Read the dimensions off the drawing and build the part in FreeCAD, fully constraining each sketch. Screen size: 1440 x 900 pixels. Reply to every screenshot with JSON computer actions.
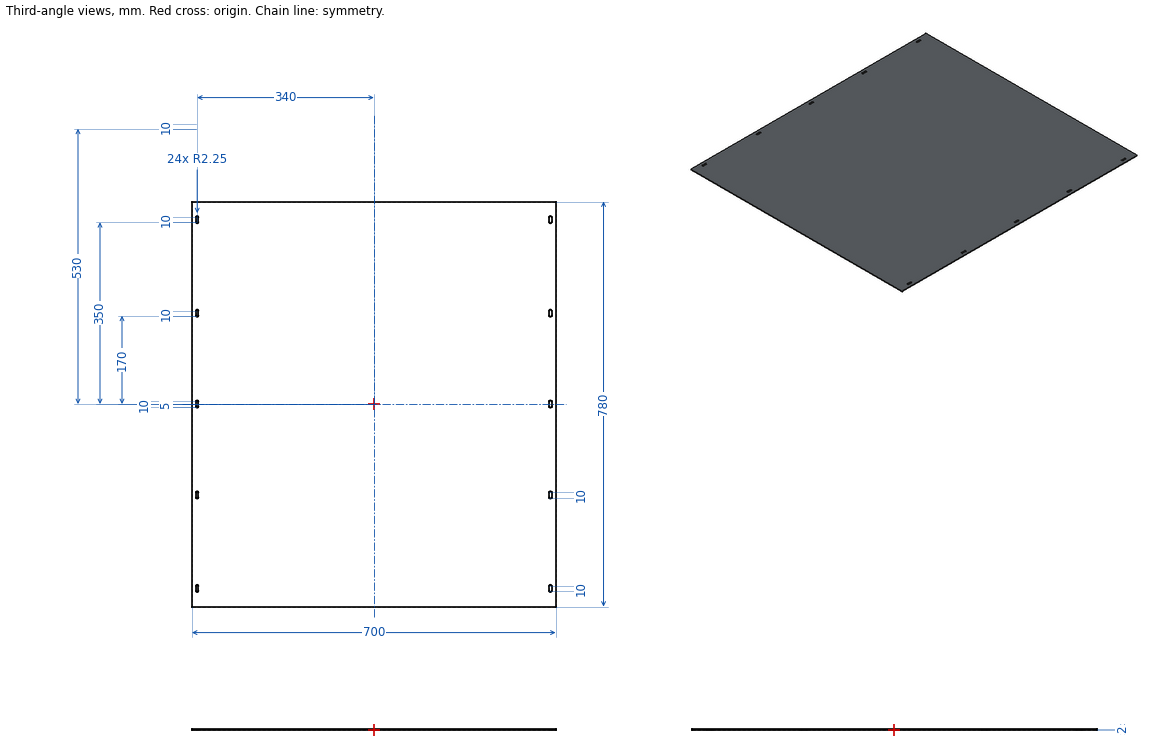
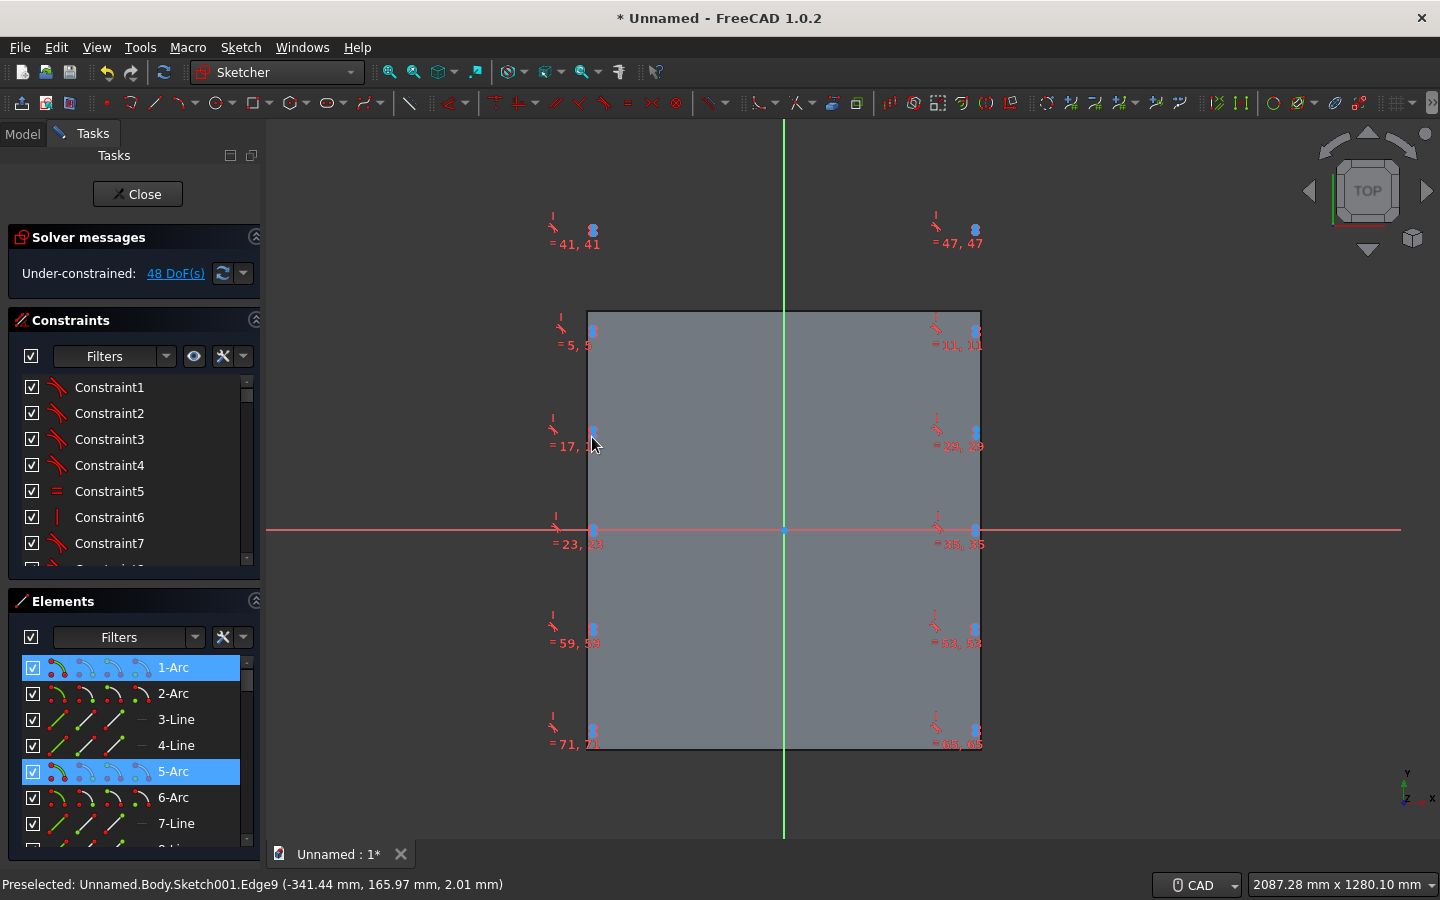
{"action": "scroll", "coordinate": [592, 534], "scroll_direction": "up", "scroll_amount": 13}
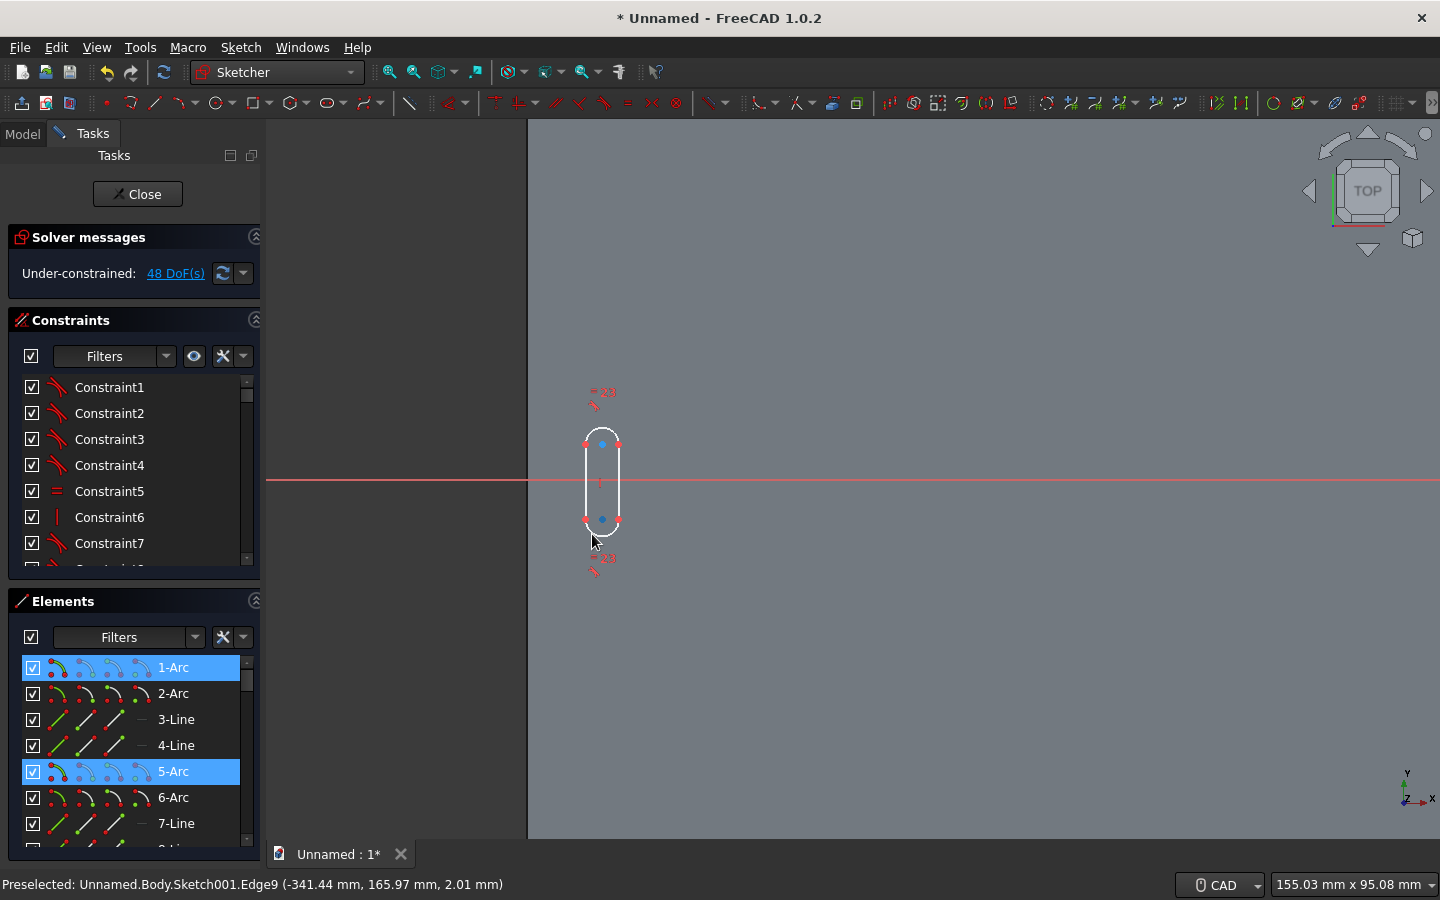
{"action": "left_click", "coordinate": [593, 533]}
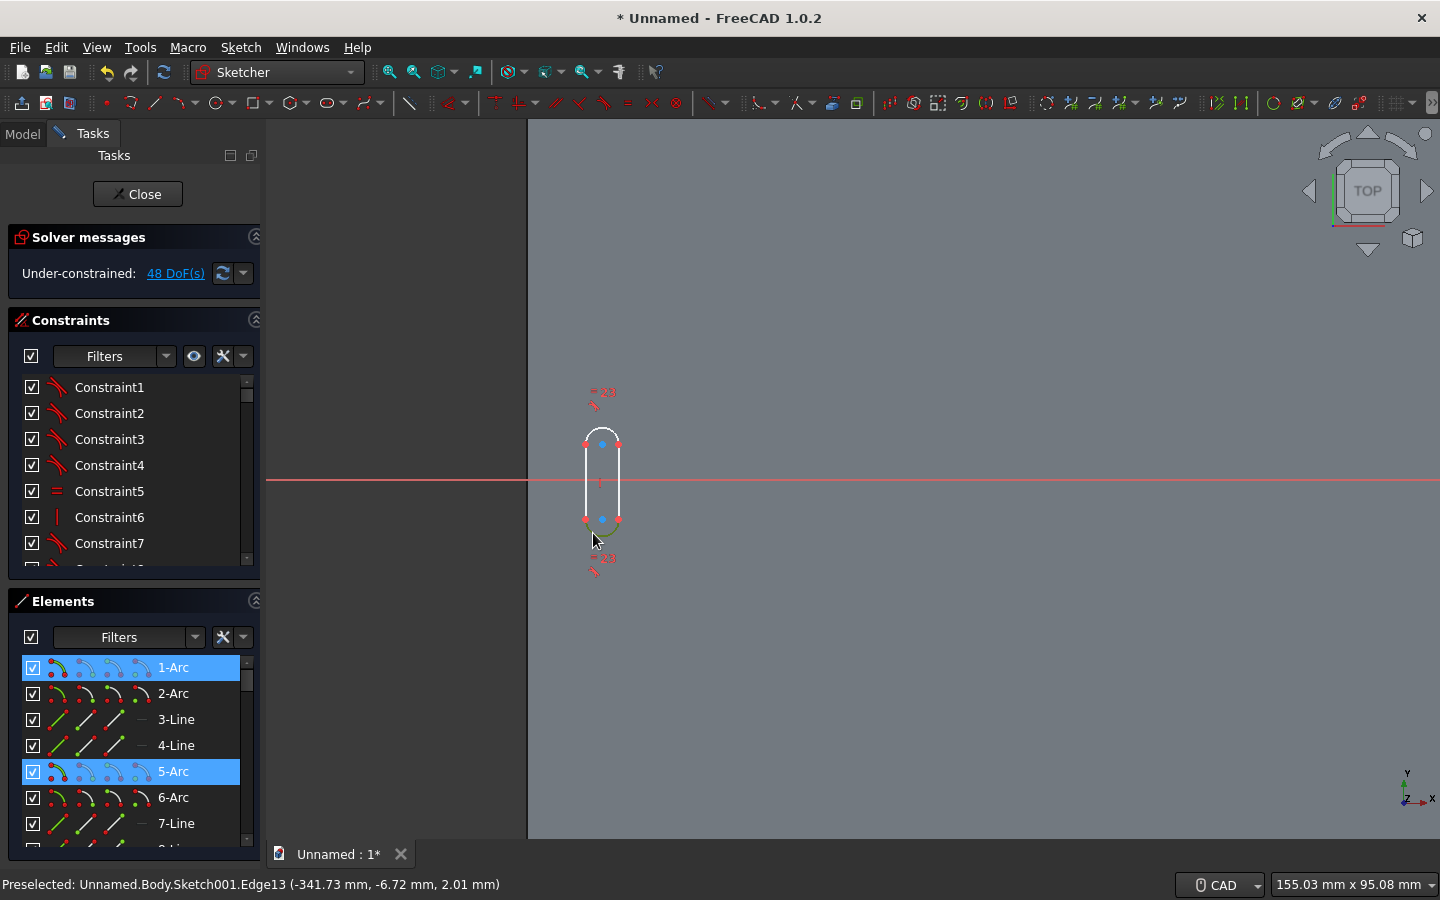
{"action": "scroll", "coordinate": [592, 534], "scroll_direction": "down", "scroll_amount": 13}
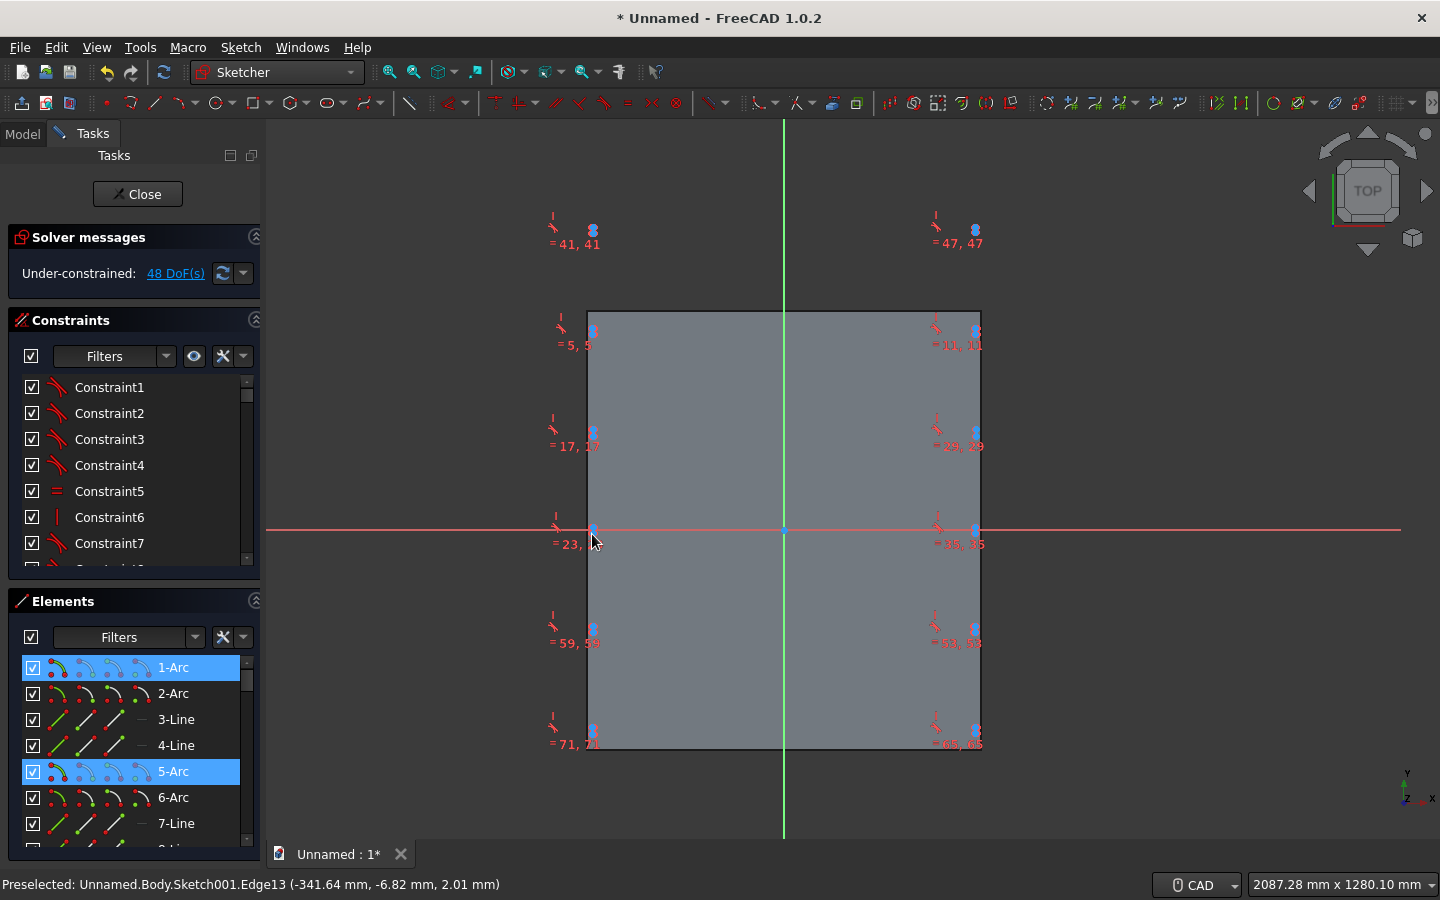
{"action": "scroll", "coordinate": [976, 437], "scroll_direction": "up", "scroll_amount": 14}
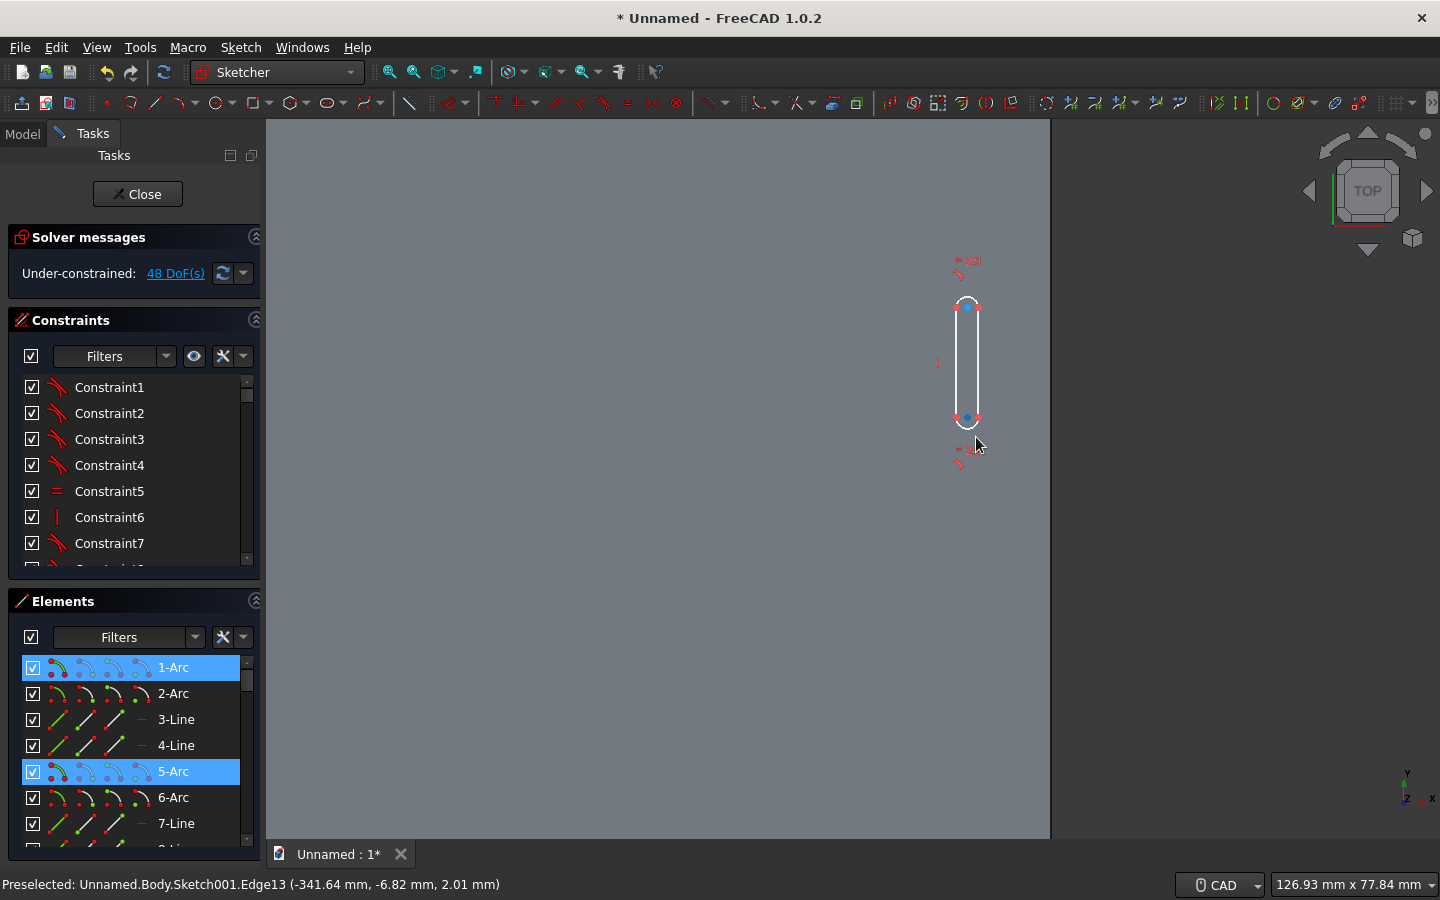
{"action": "left_click", "coordinate": [967, 429]}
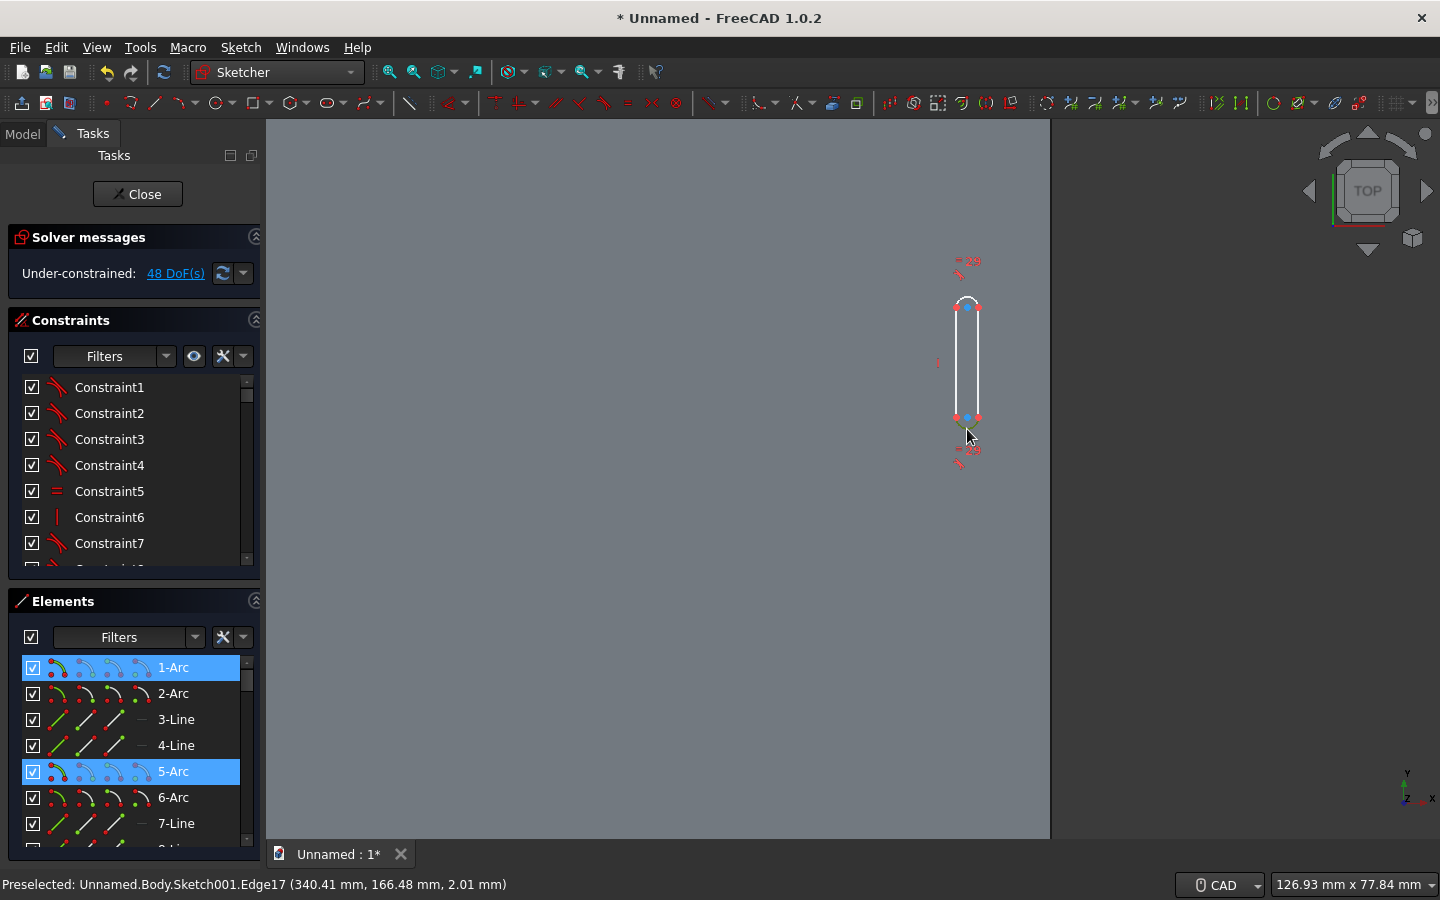
{"action": "scroll", "coordinate": [977, 437], "scroll_direction": "down", "scroll_amount": 14}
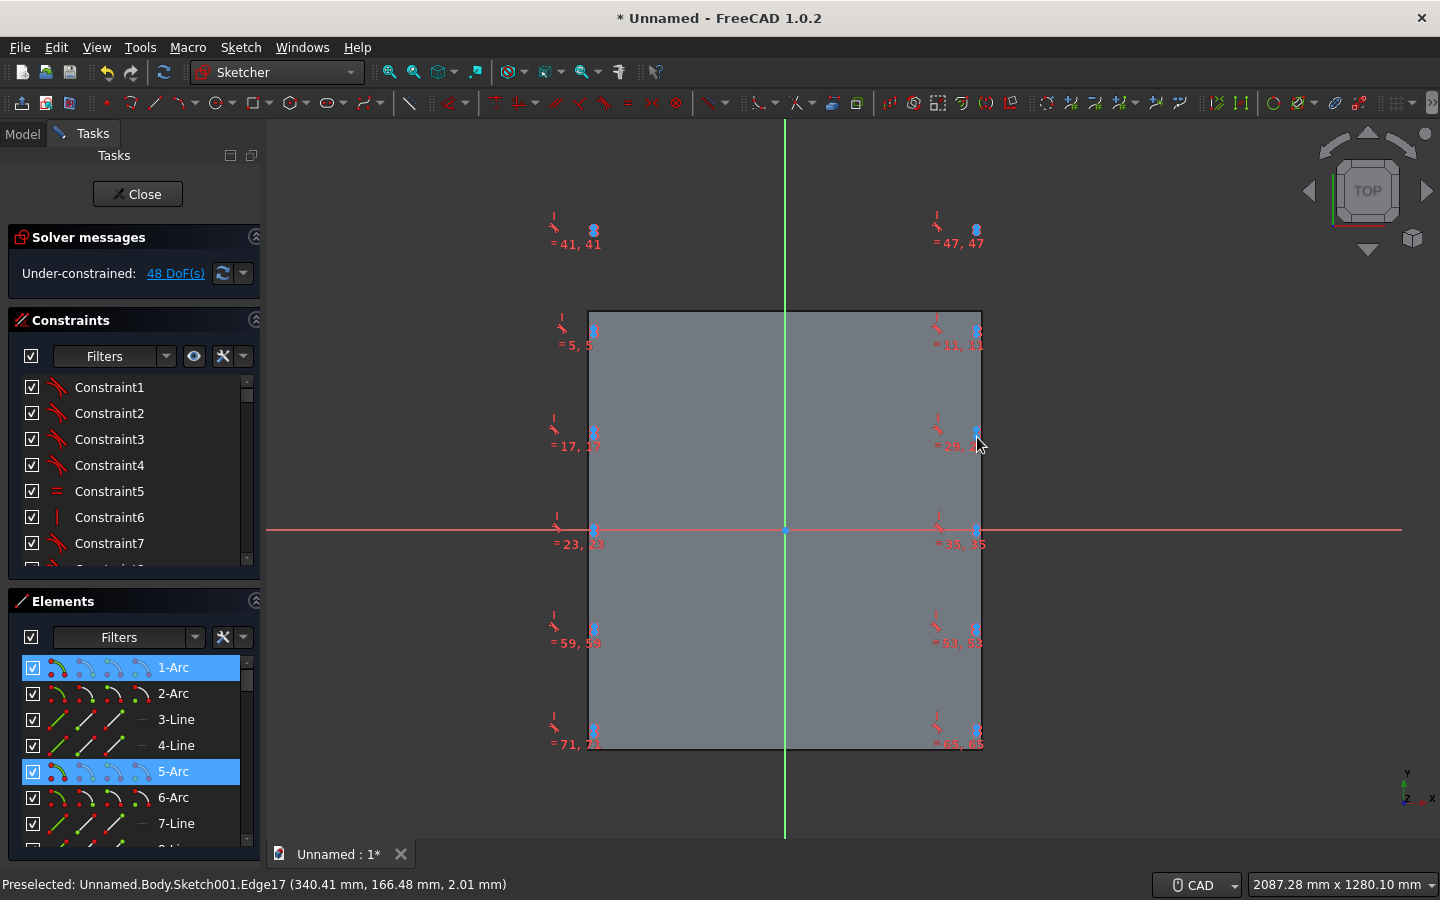
{"action": "scroll", "coordinate": [976, 535], "scroll_direction": "up", "scroll_amount": 13}